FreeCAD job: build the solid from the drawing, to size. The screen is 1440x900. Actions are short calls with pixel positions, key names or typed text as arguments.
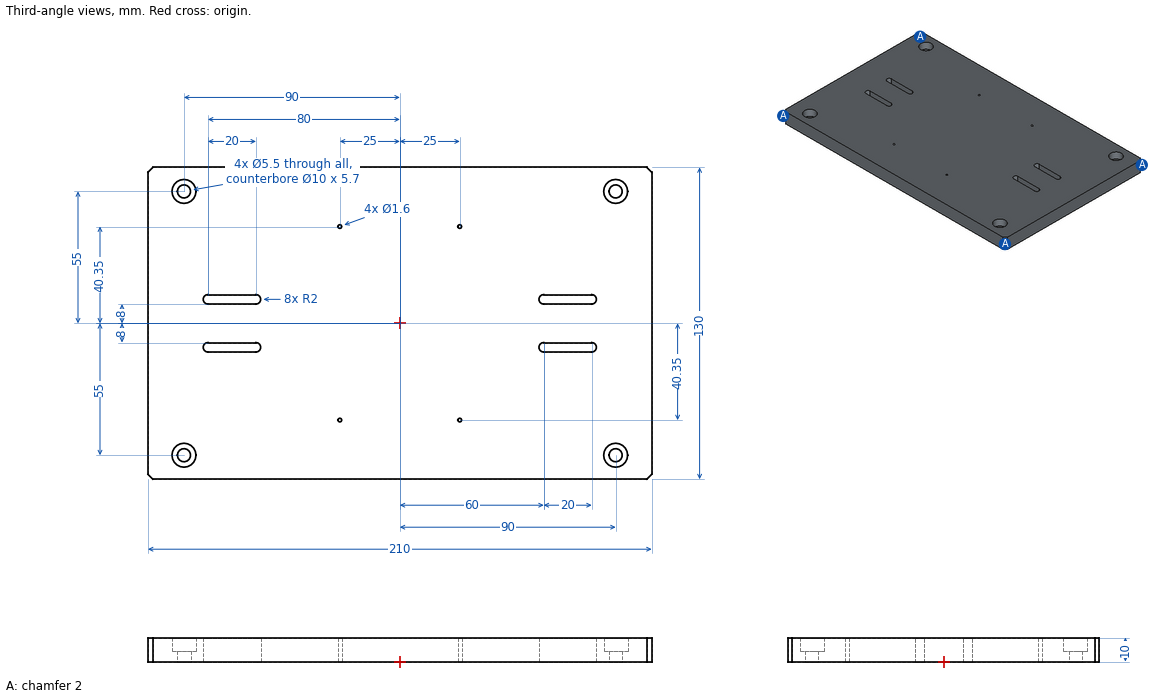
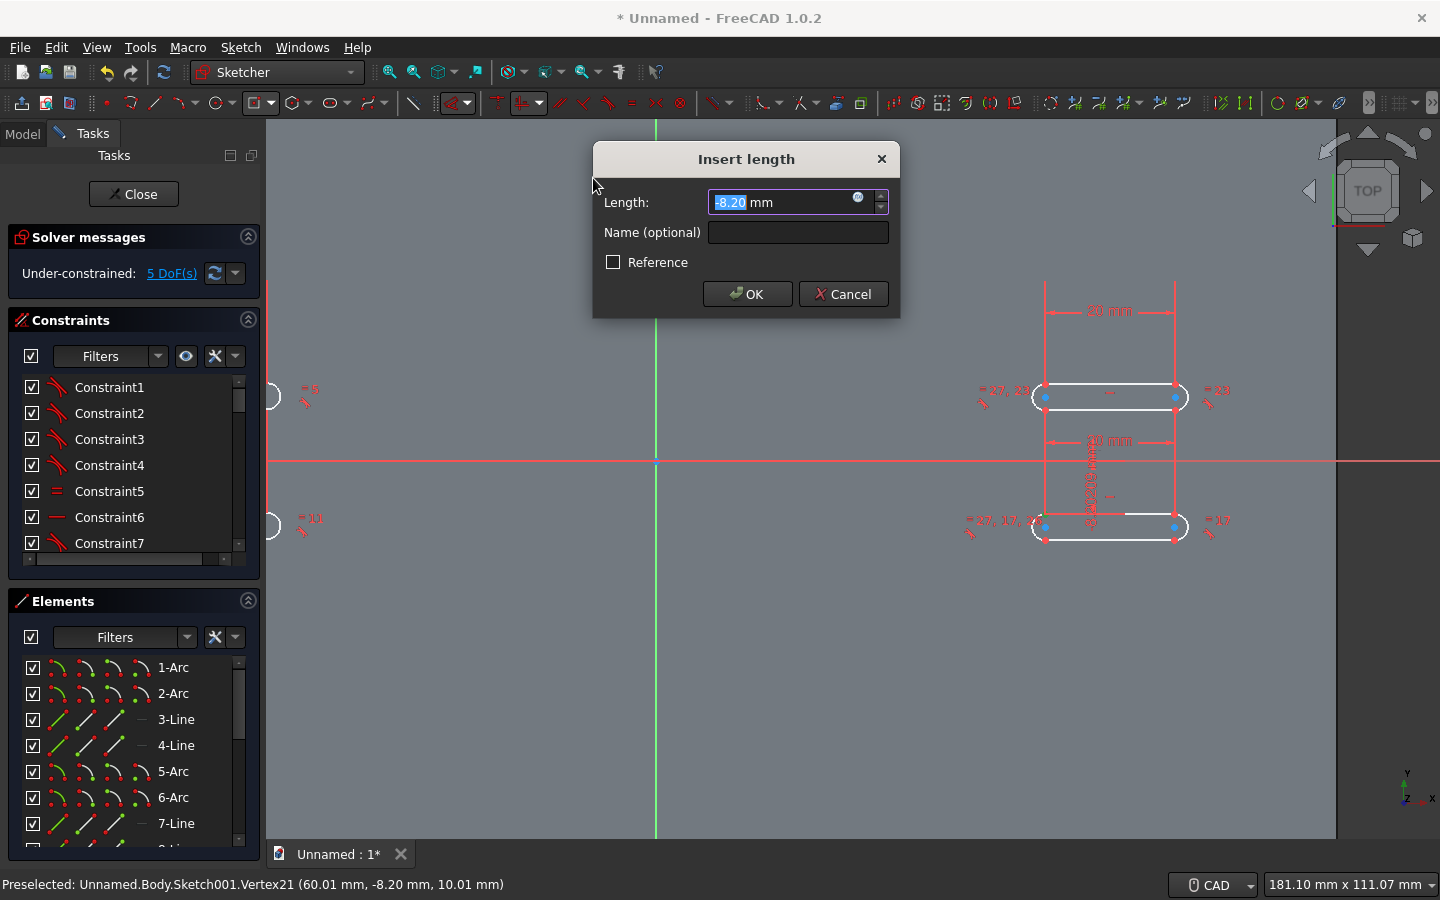
text(-8)
key(Return)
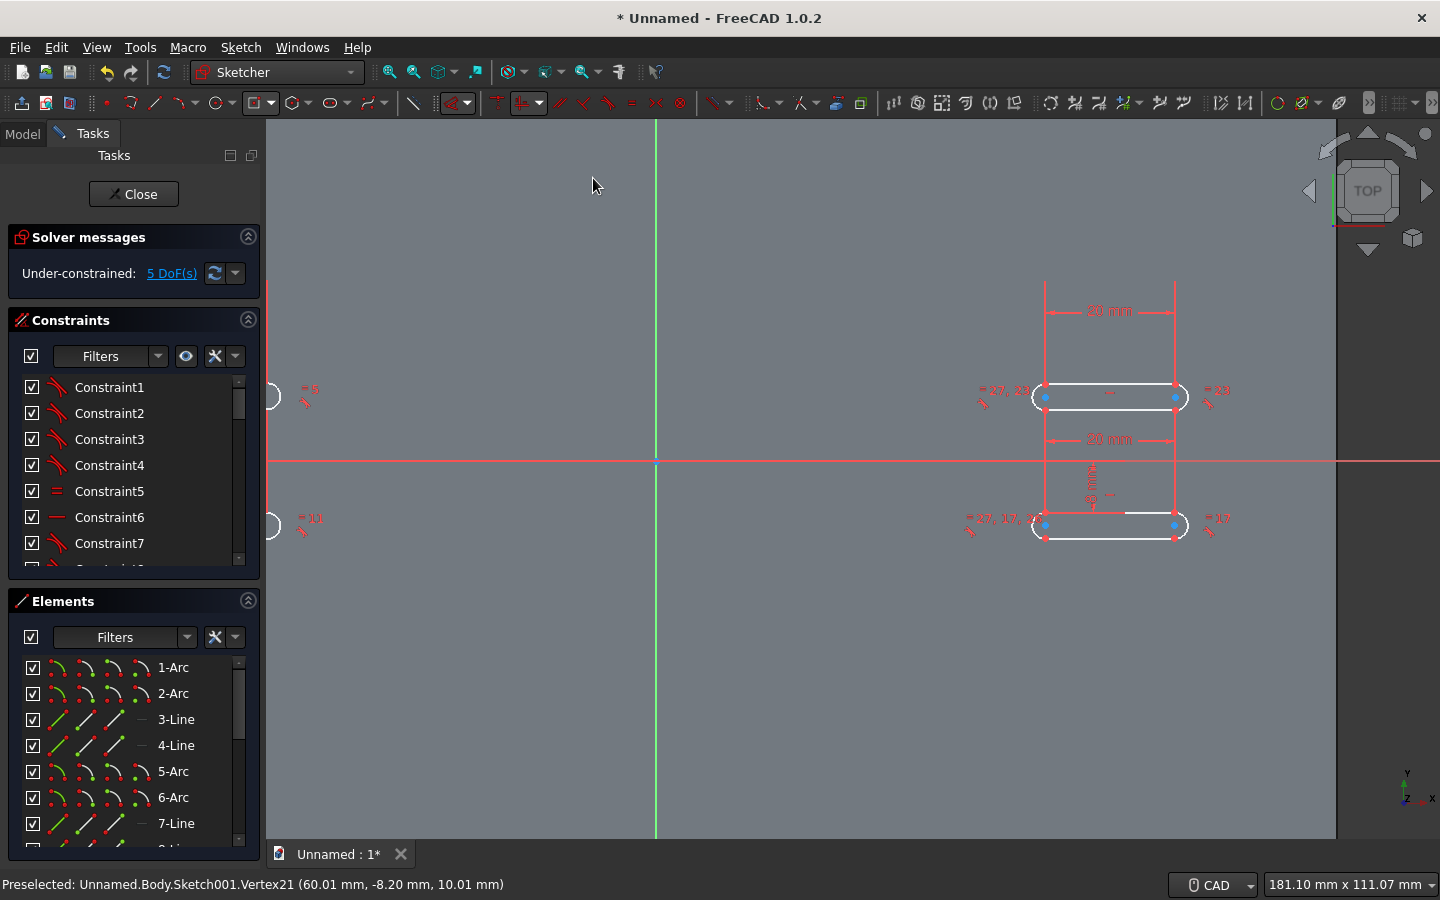
click(1045, 410)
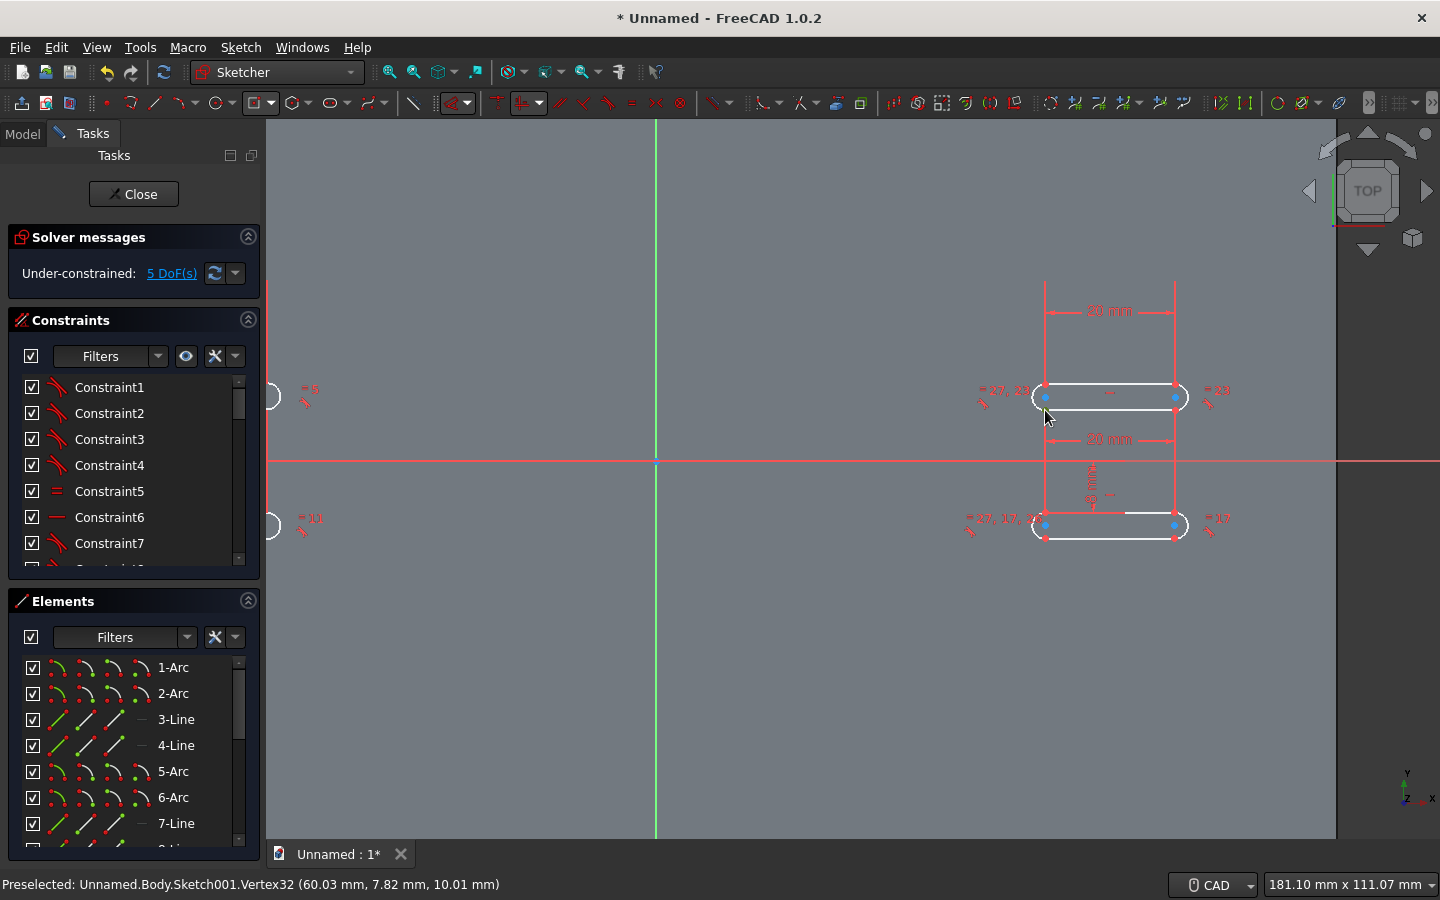
click(470, 104)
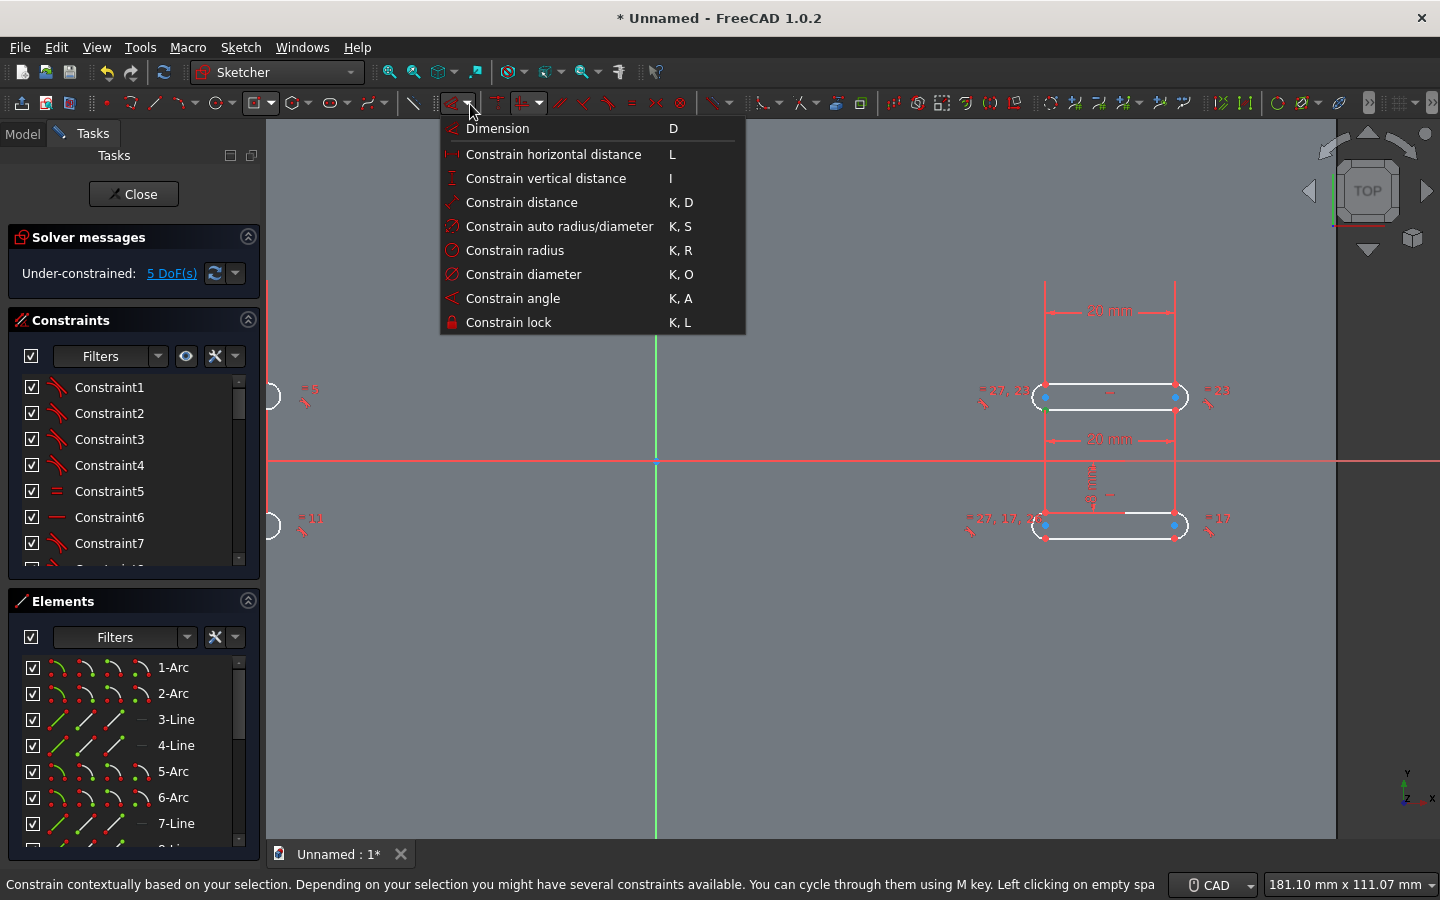
click(593, 178)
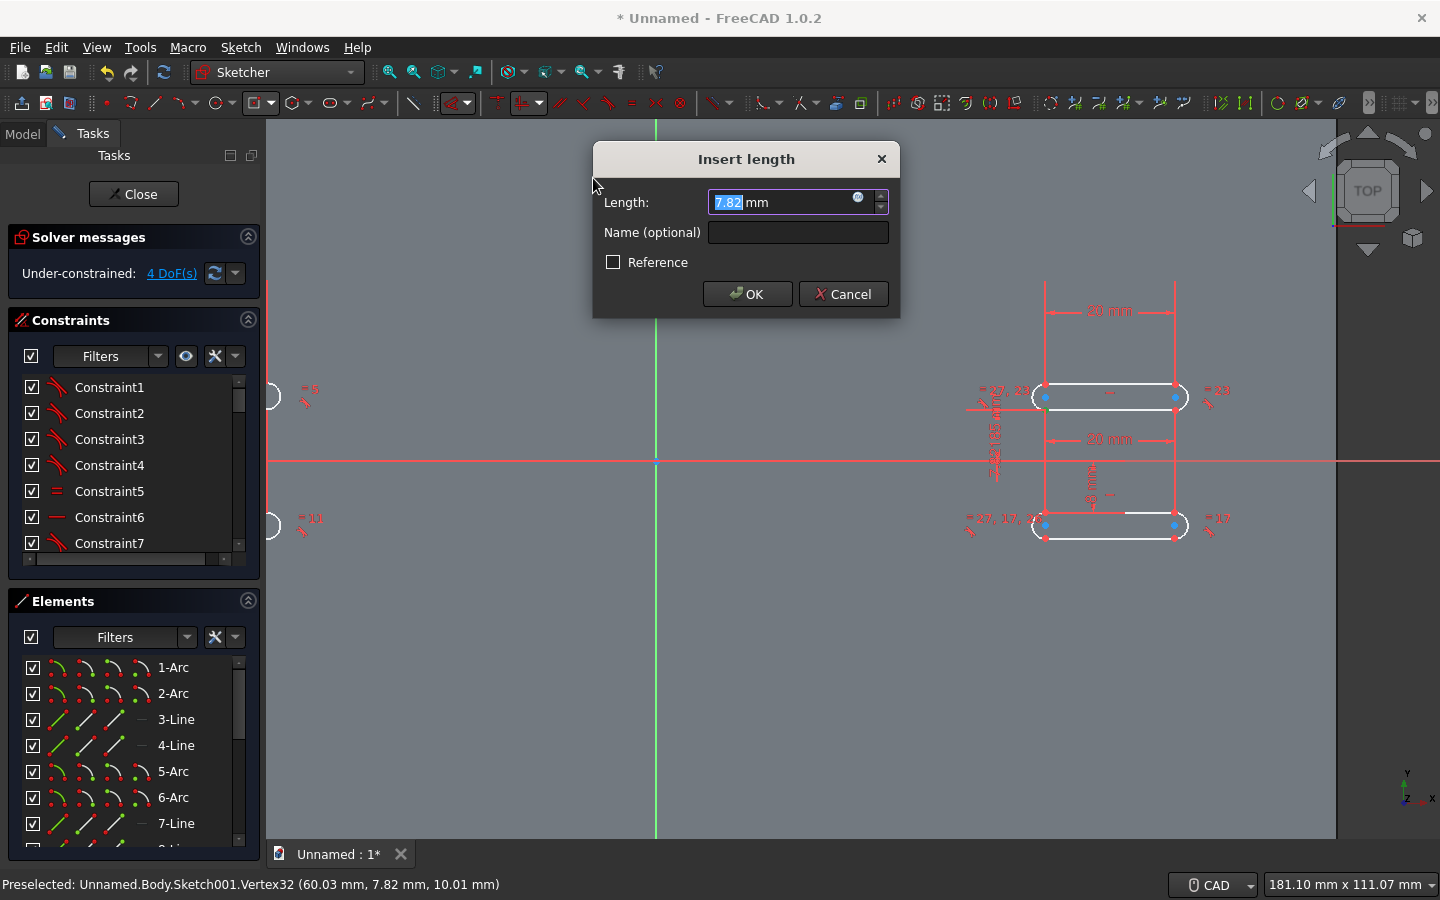
text(8)
key(Return)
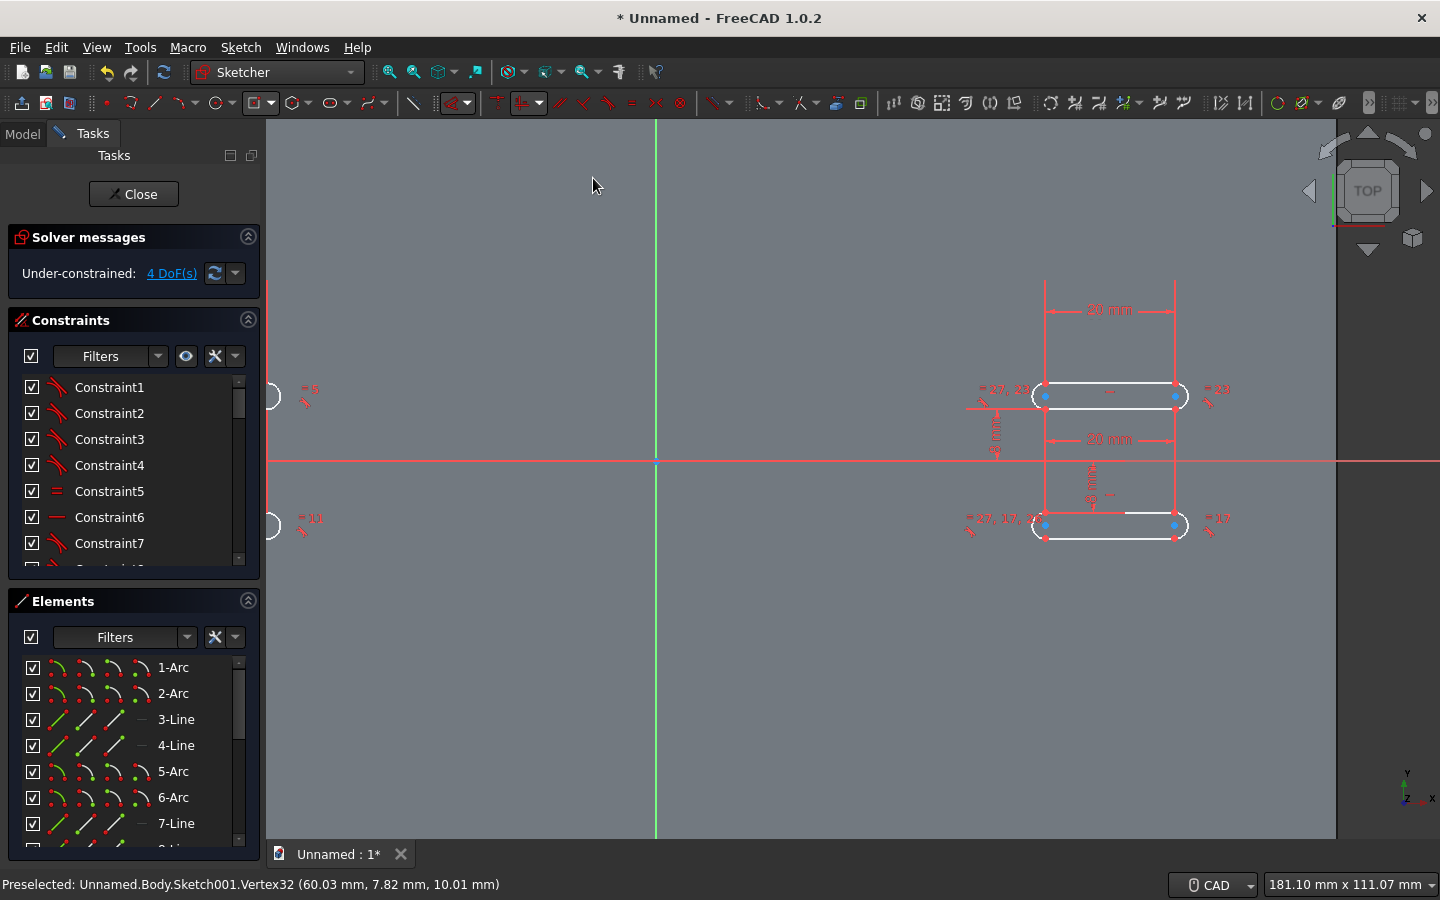
scroll(1045, 515, down, 2)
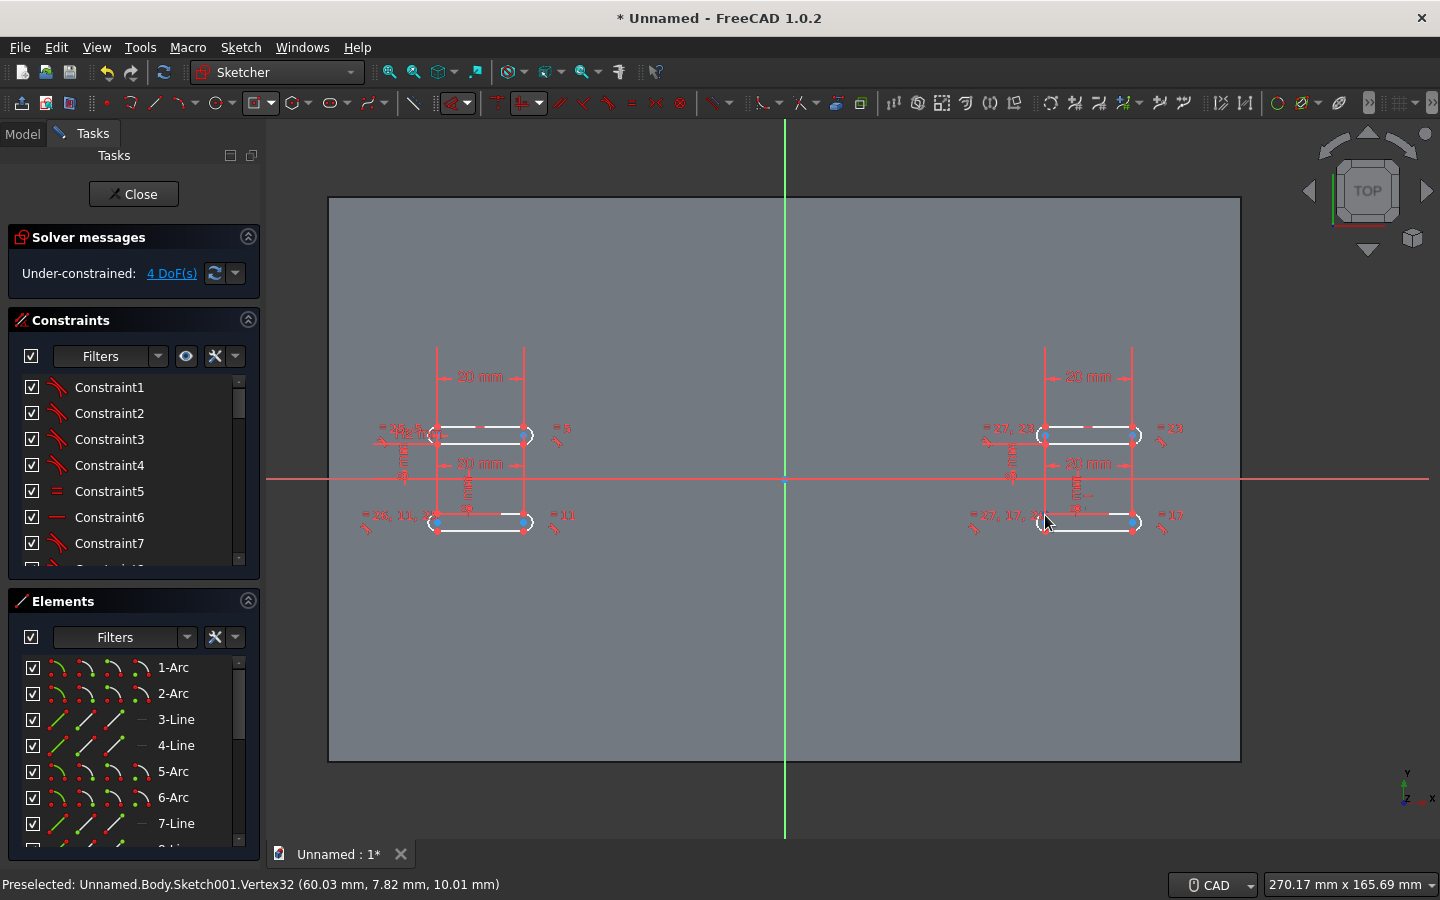
scroll(437, 427, up, 2)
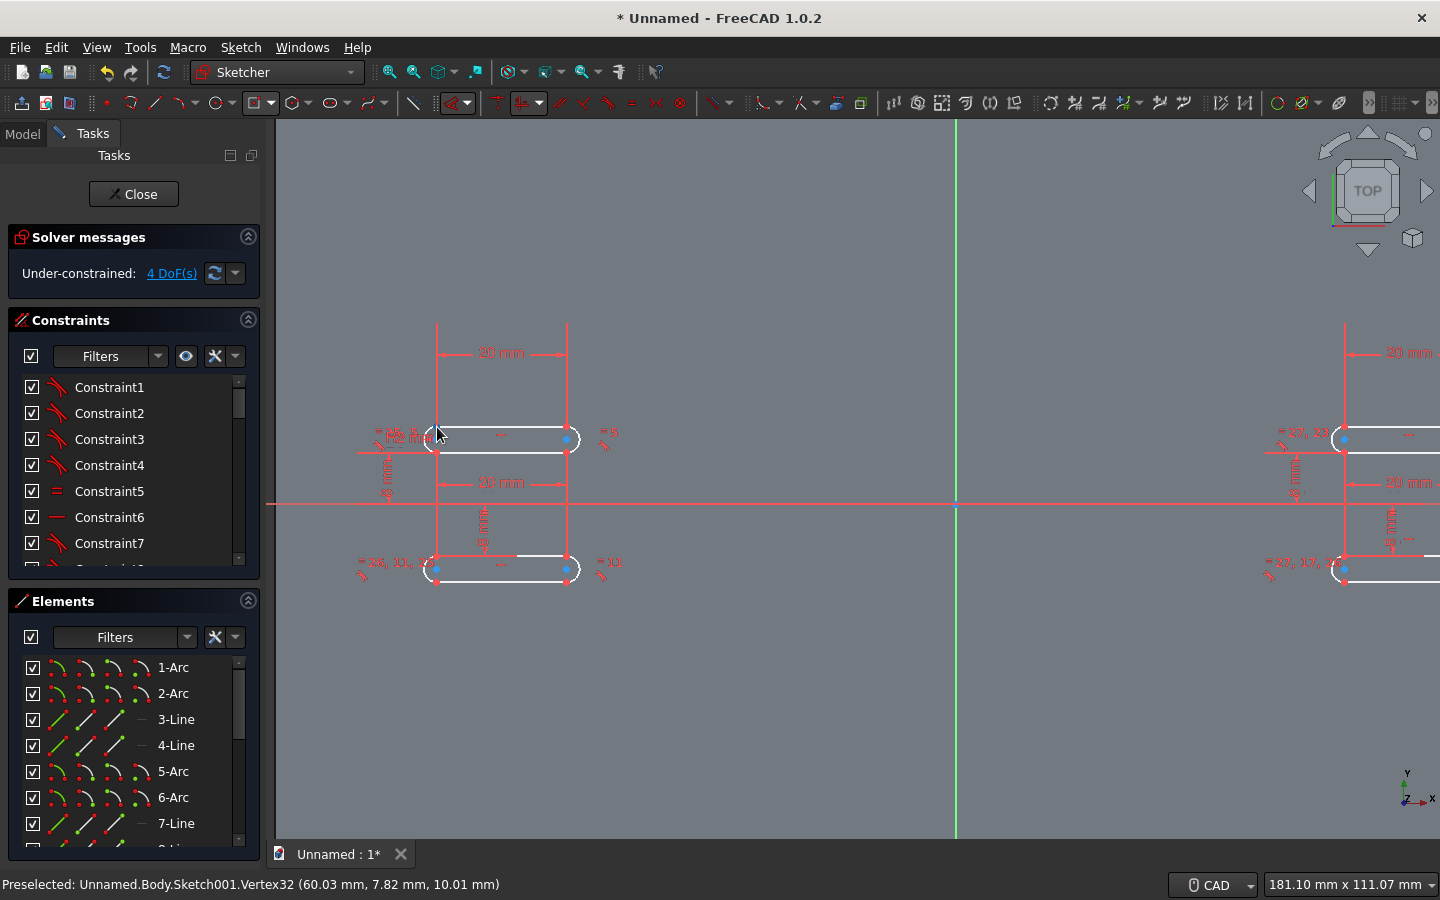
click(437, 427)